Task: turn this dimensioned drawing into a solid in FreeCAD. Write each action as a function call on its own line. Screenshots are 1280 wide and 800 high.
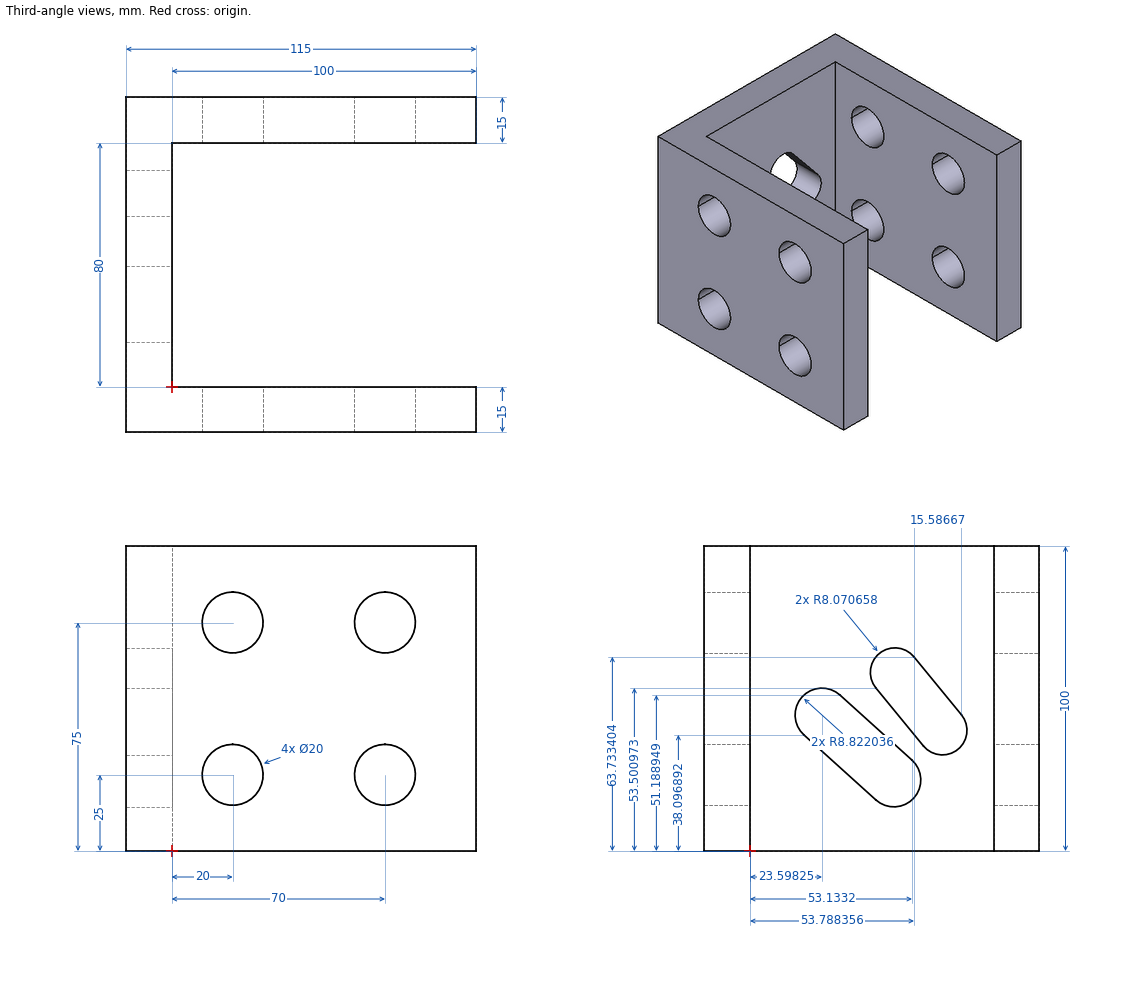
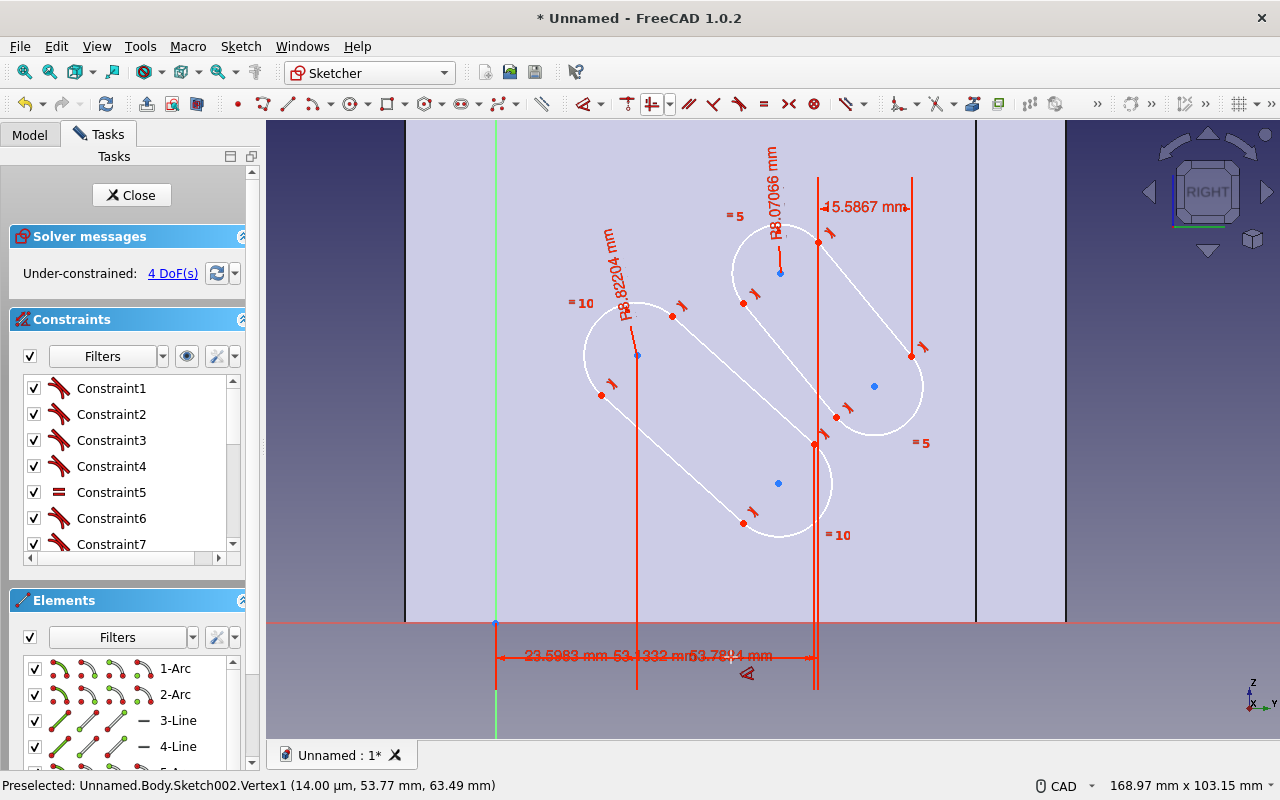
click(818, 242)
click(462, 433)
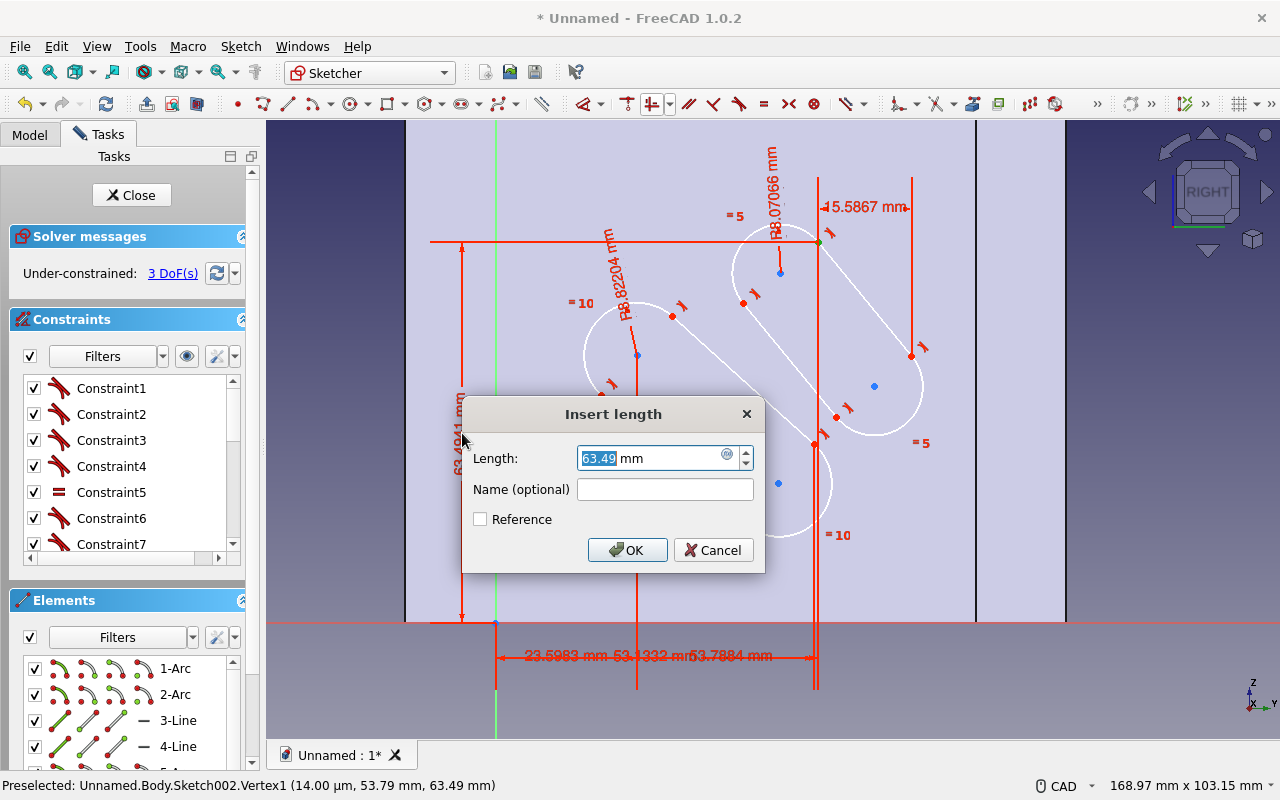
text(63.733404)
key(Return)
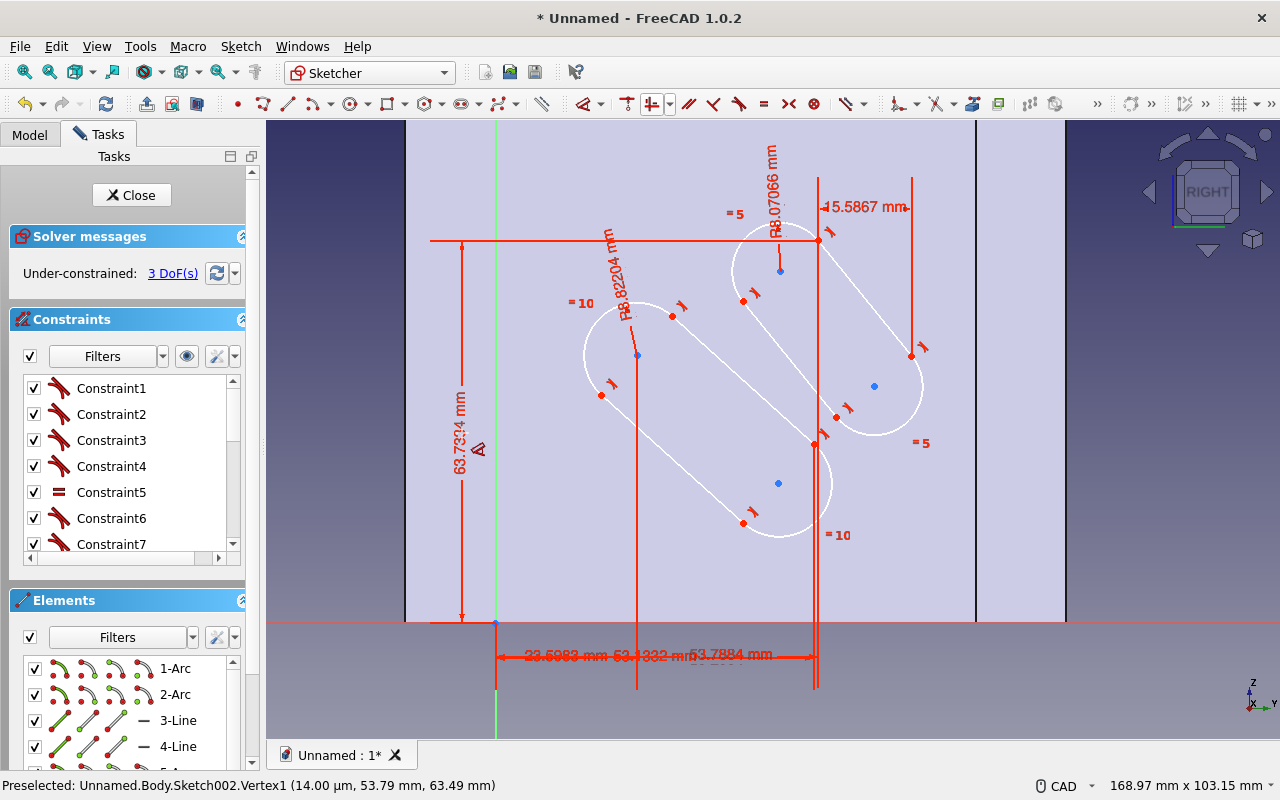
click(743, 302)
click(462, 463)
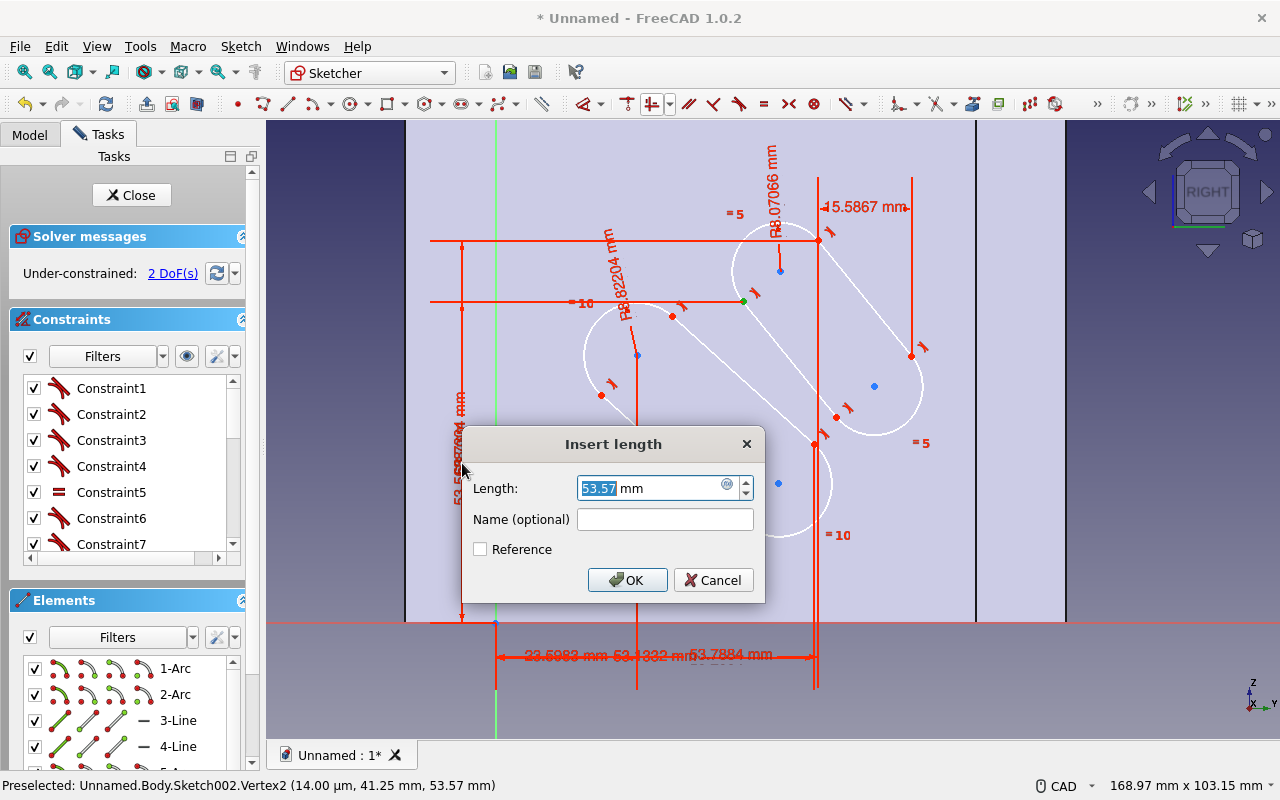
text(53.500973)
key(Return)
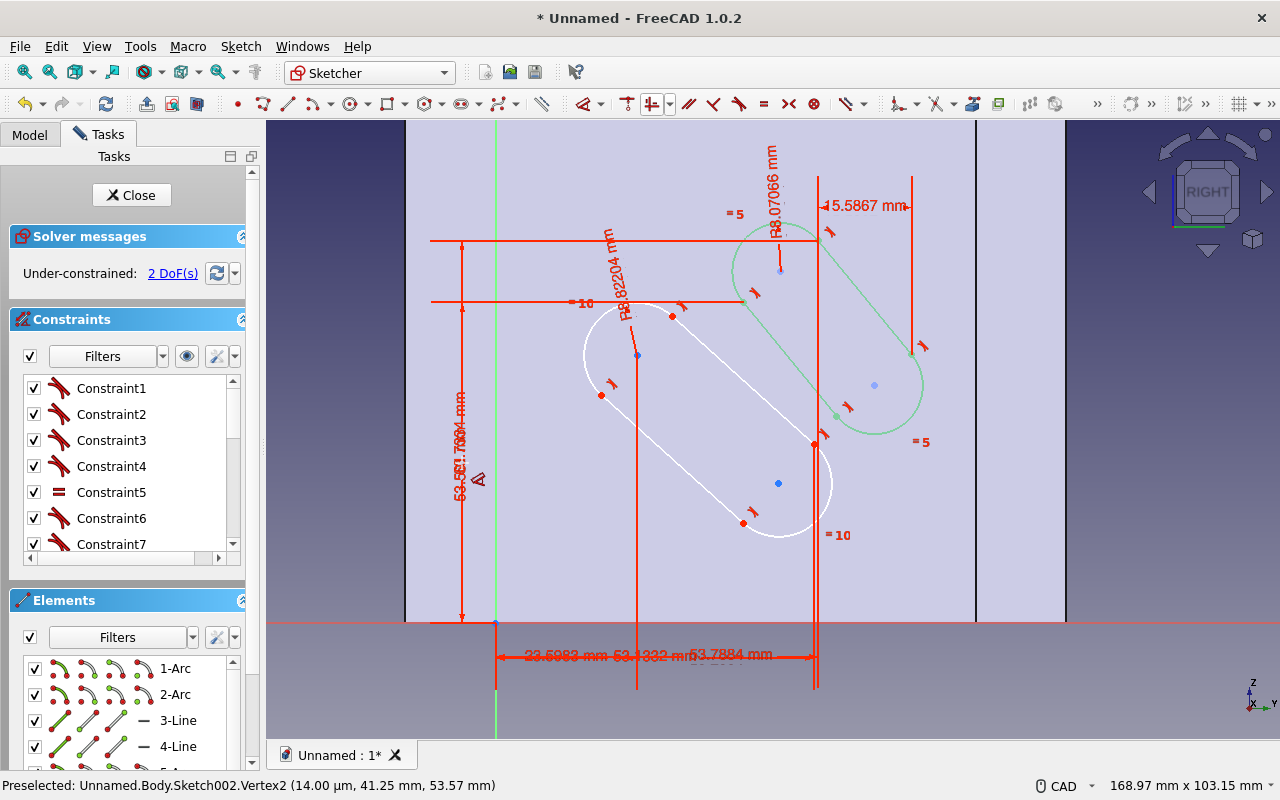
click(673, 317)
click(462, 399)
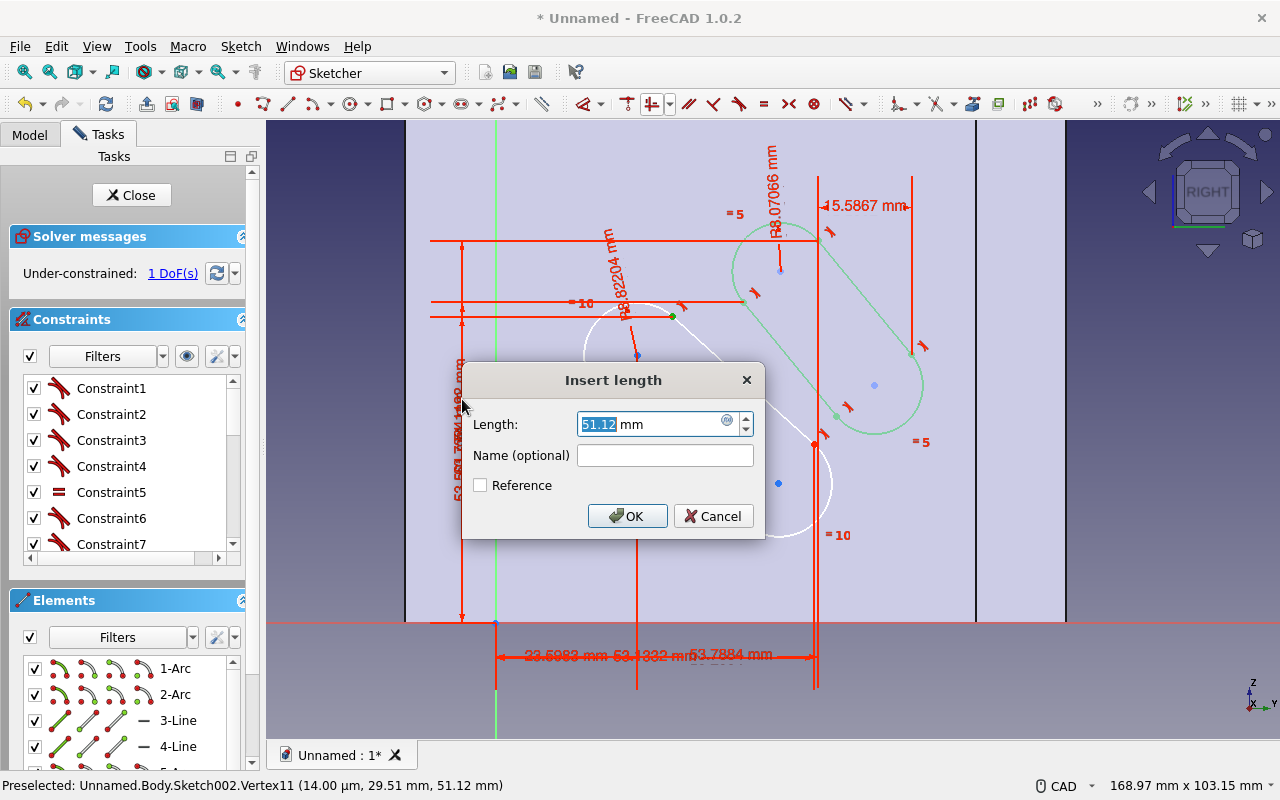
text(51.188949)
key(Return)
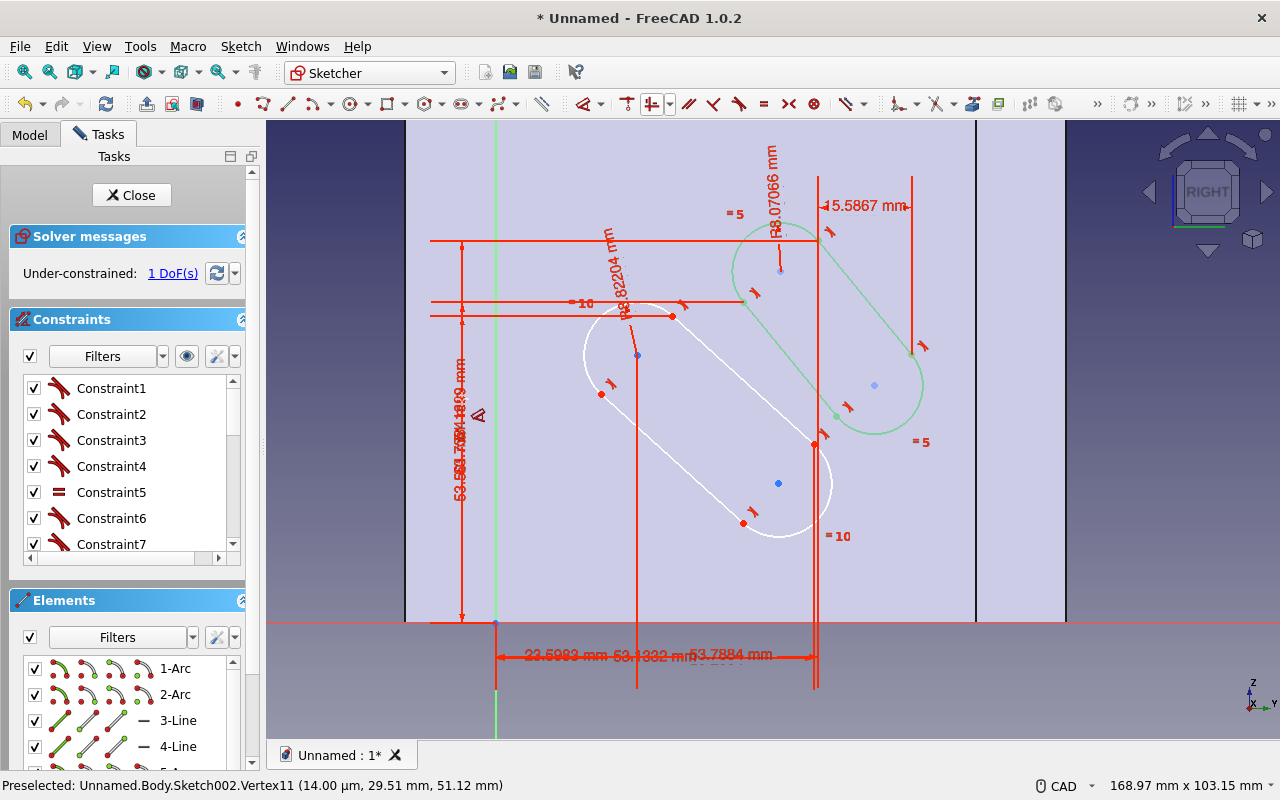
click(602, 395)
click(462, 509)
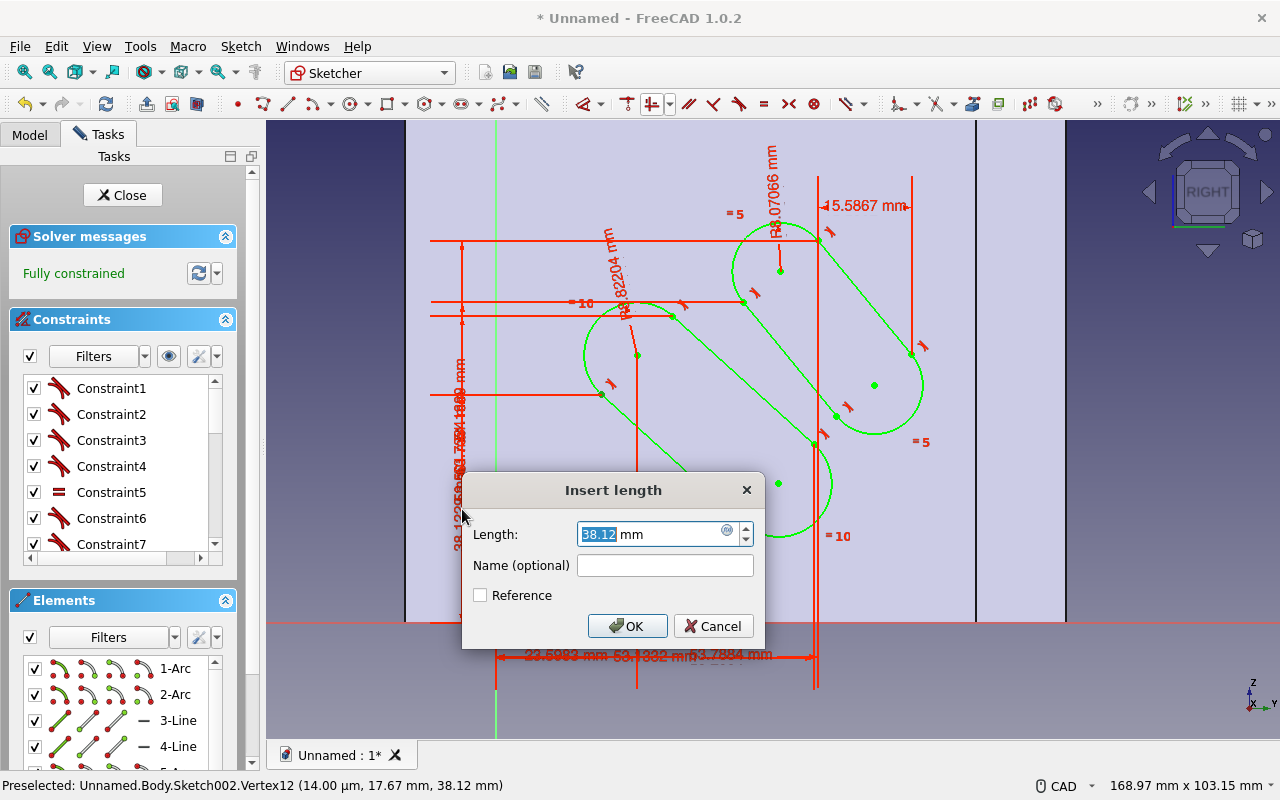
text(38.096892)
key(Return)
key(Escape)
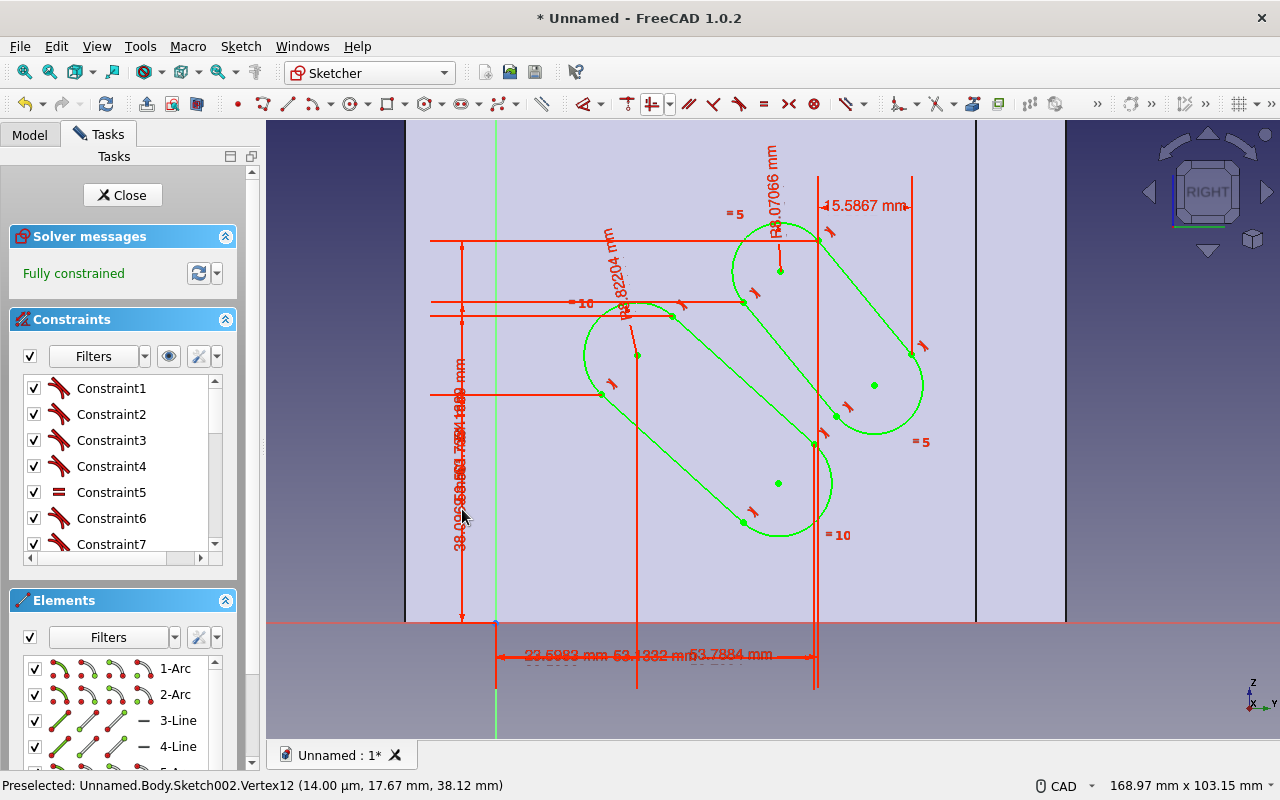
click(123, 195)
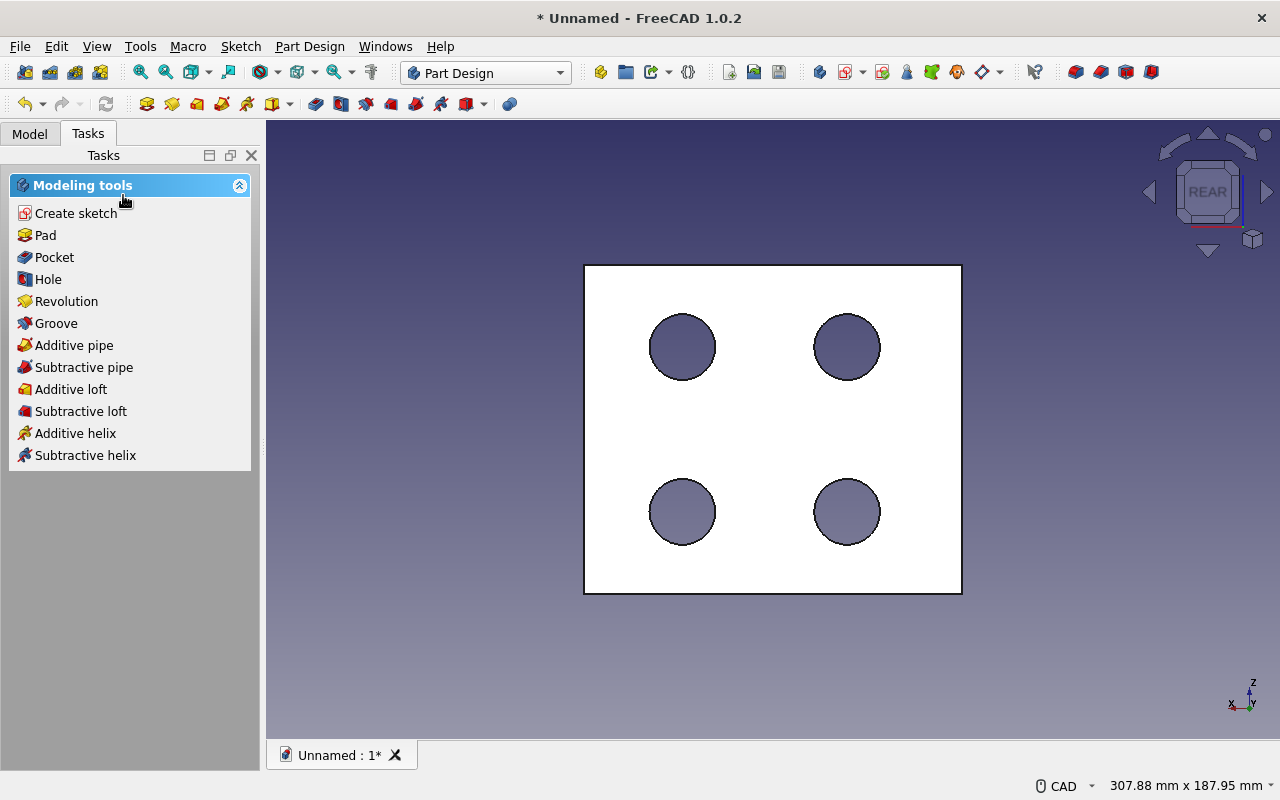
click(316, 104)